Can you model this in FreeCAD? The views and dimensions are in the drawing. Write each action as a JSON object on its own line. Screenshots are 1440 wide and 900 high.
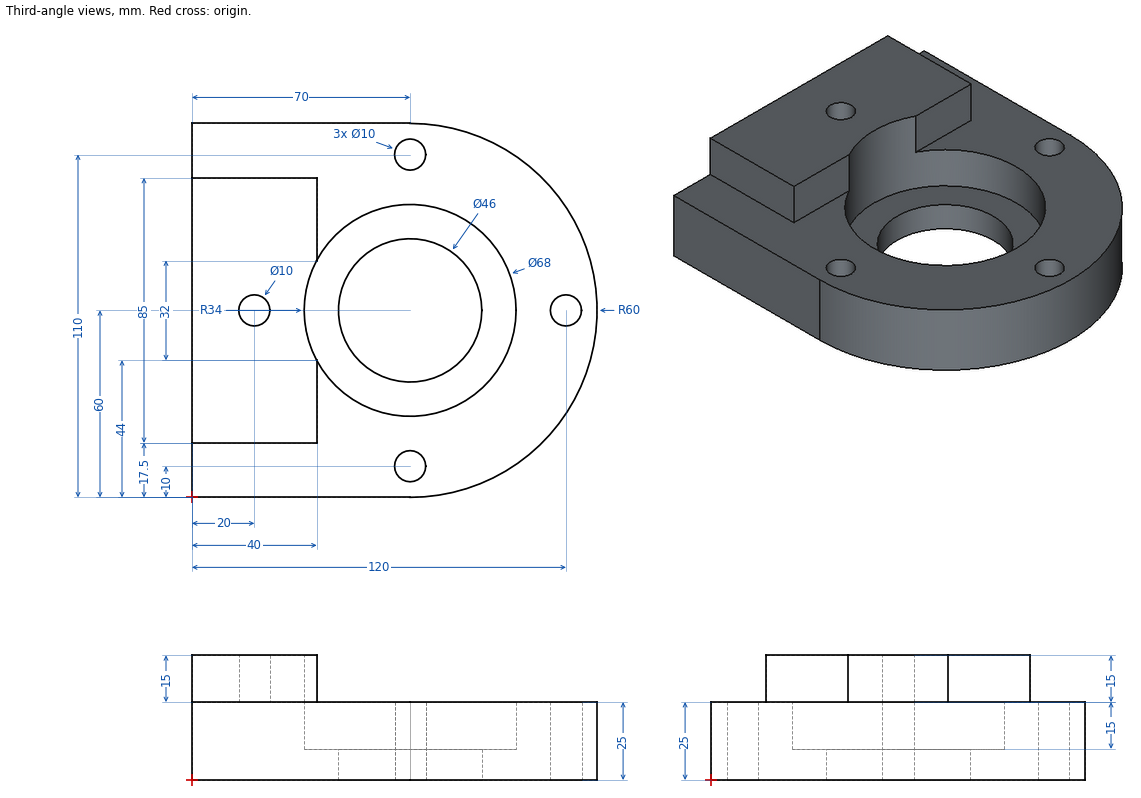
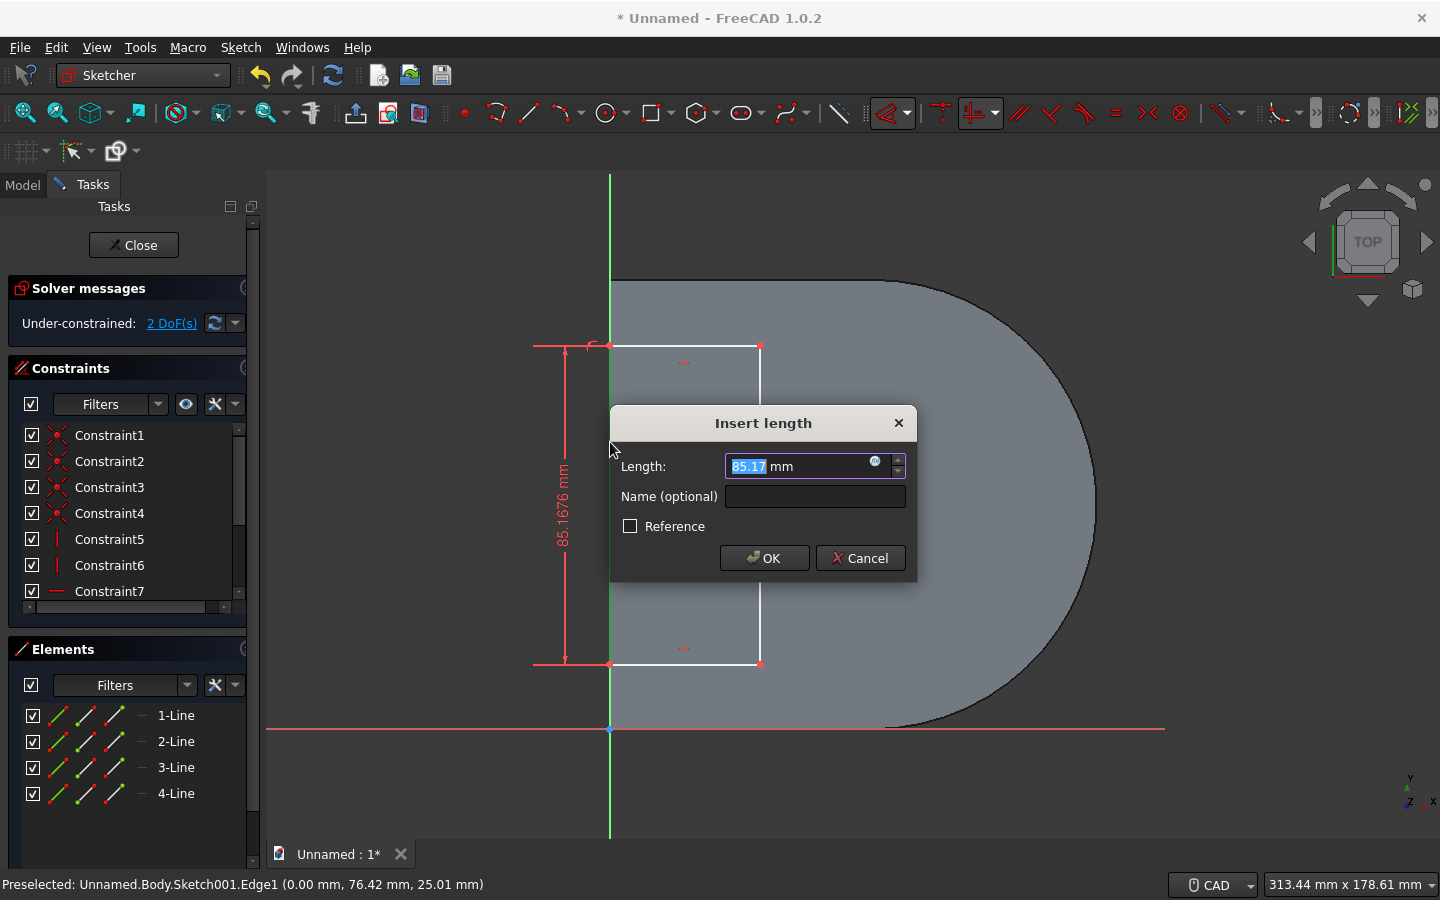
{"action": "type", "text": "85"}
{"action": "key", "text": "Return"}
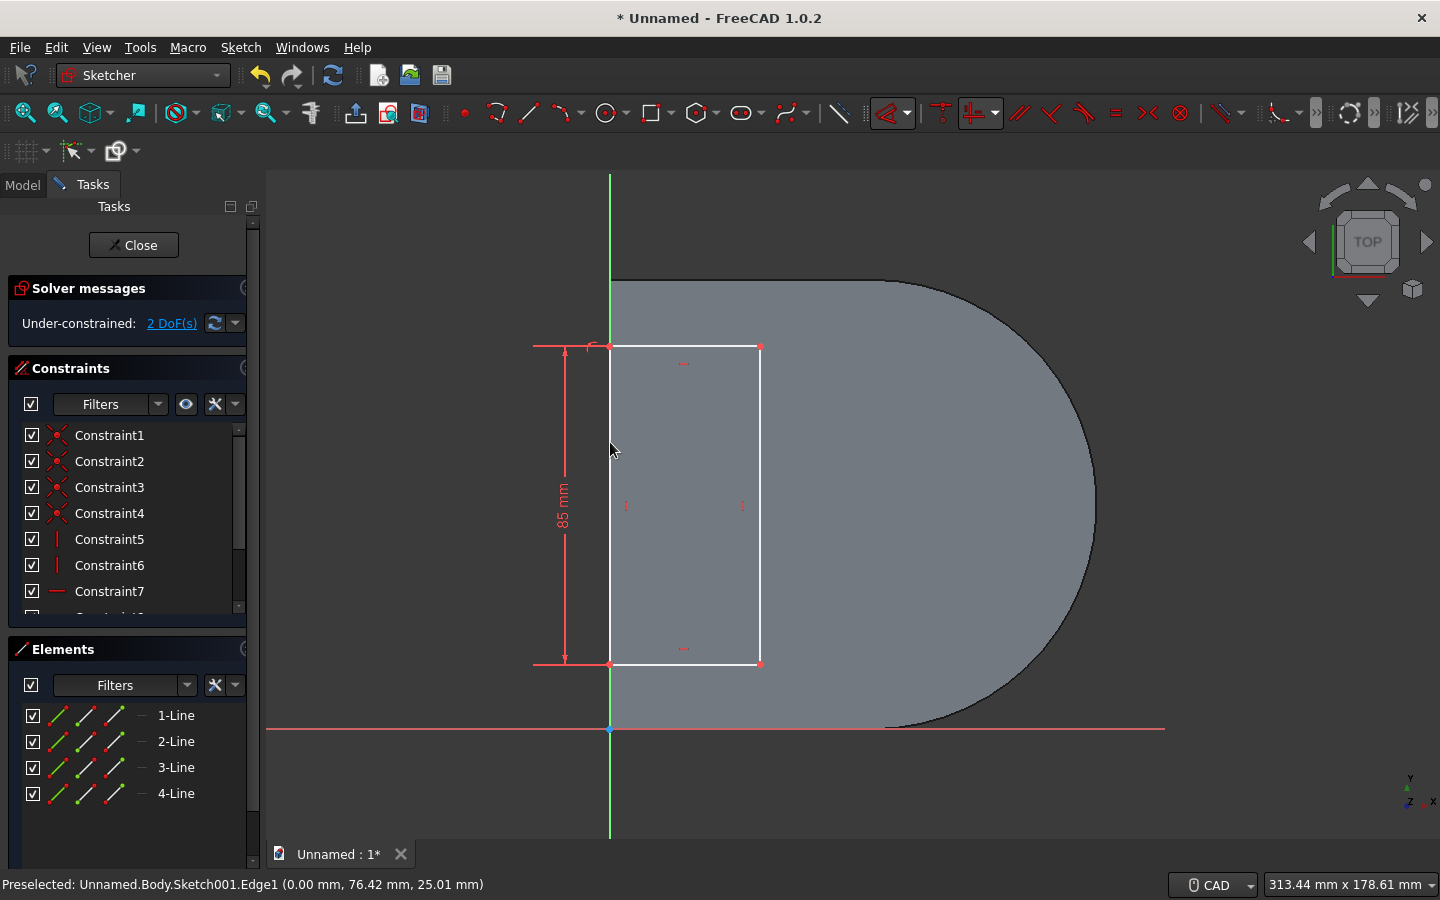
{"action": "left_click", "coordinate": [655, 665]}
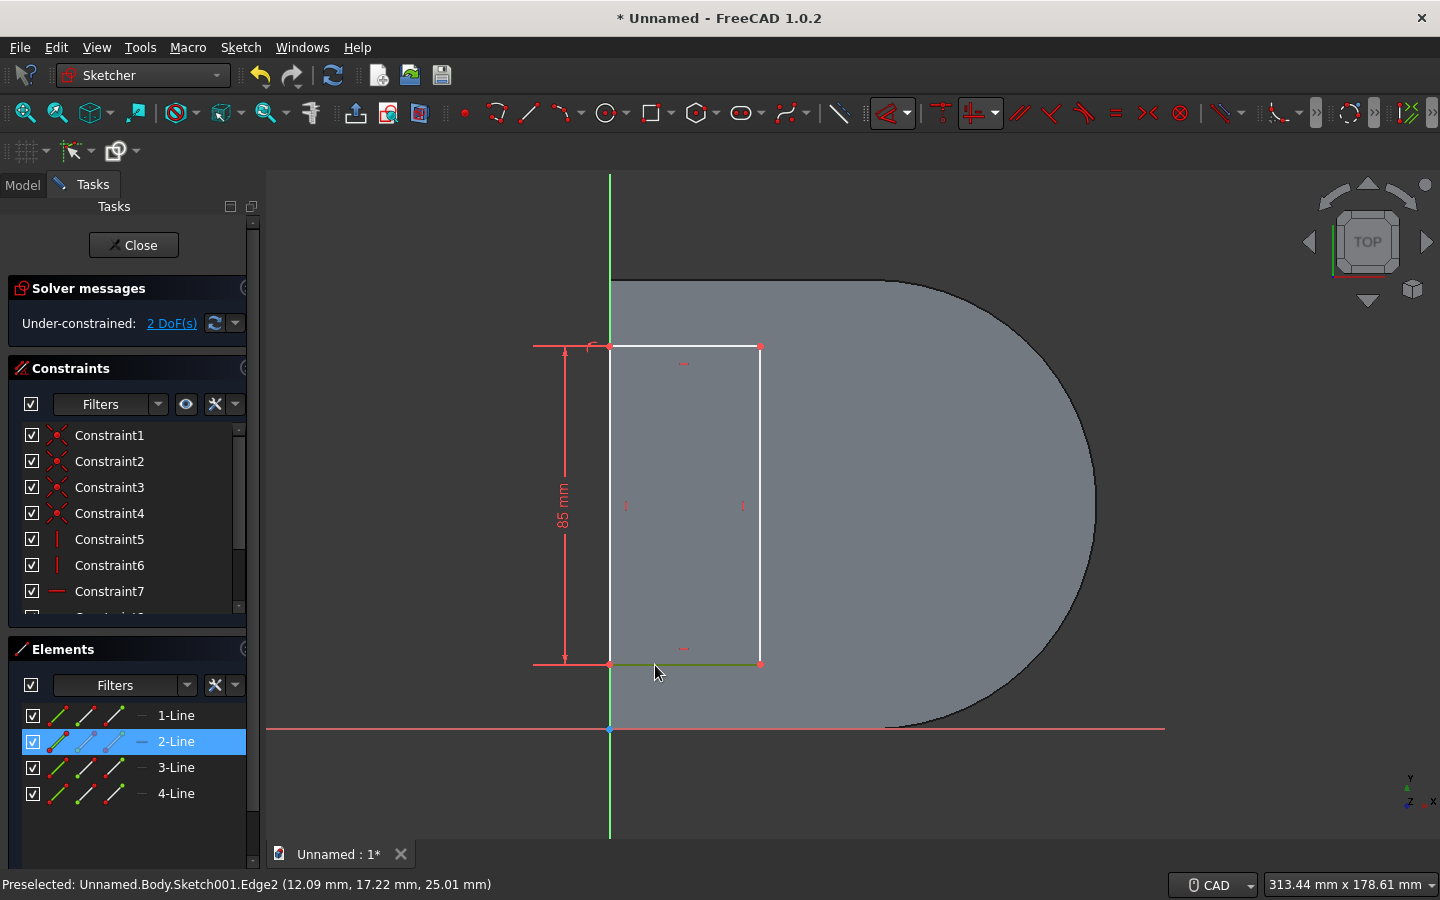
{"action": "key", "text": "l"}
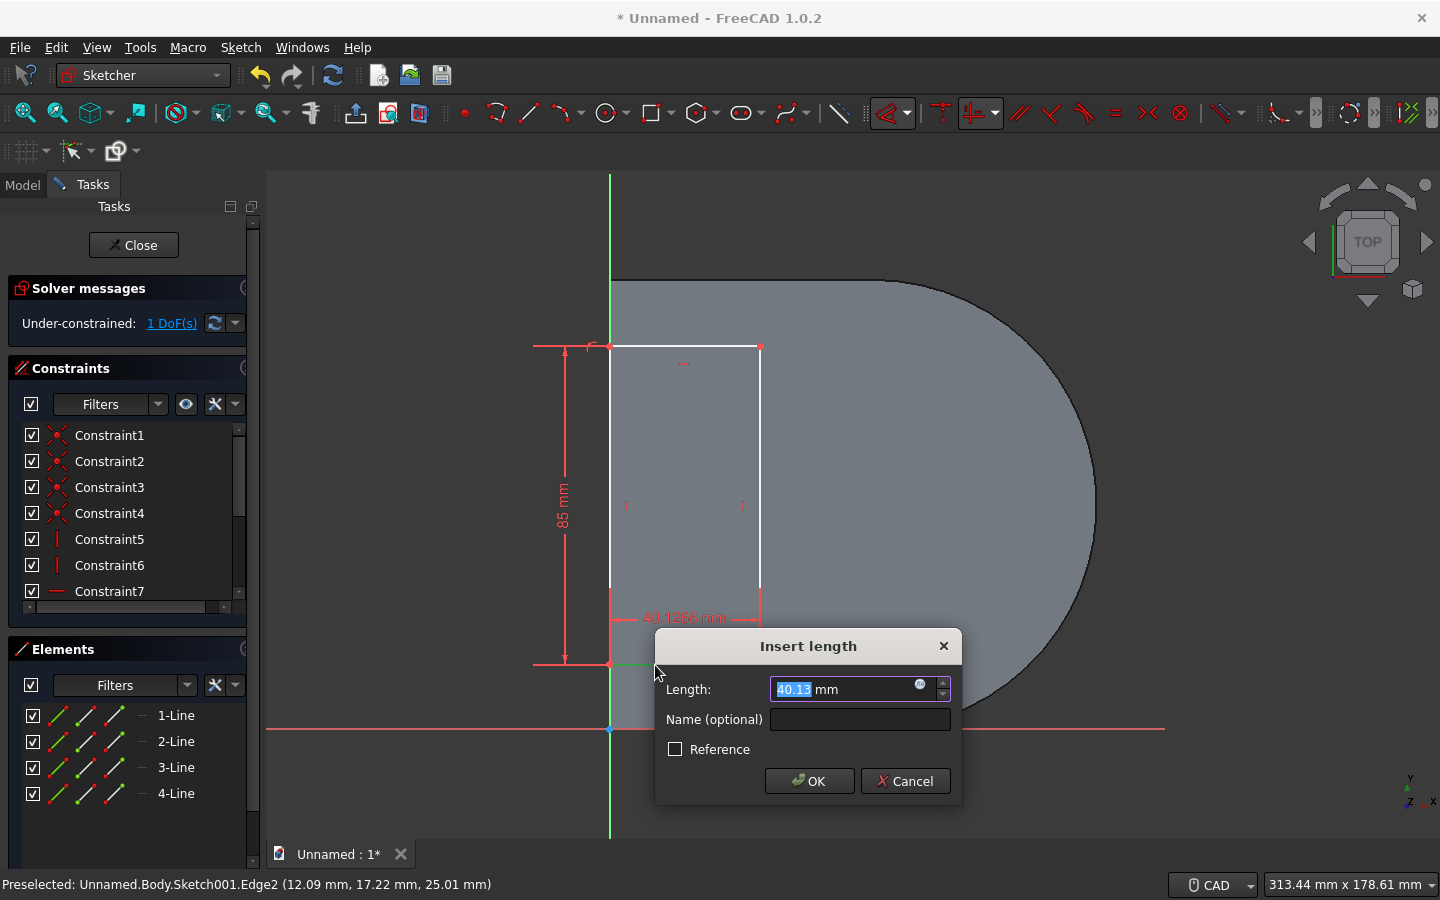
{"action": "type", "text": "40"}
{"action": "key", "text": "Return"}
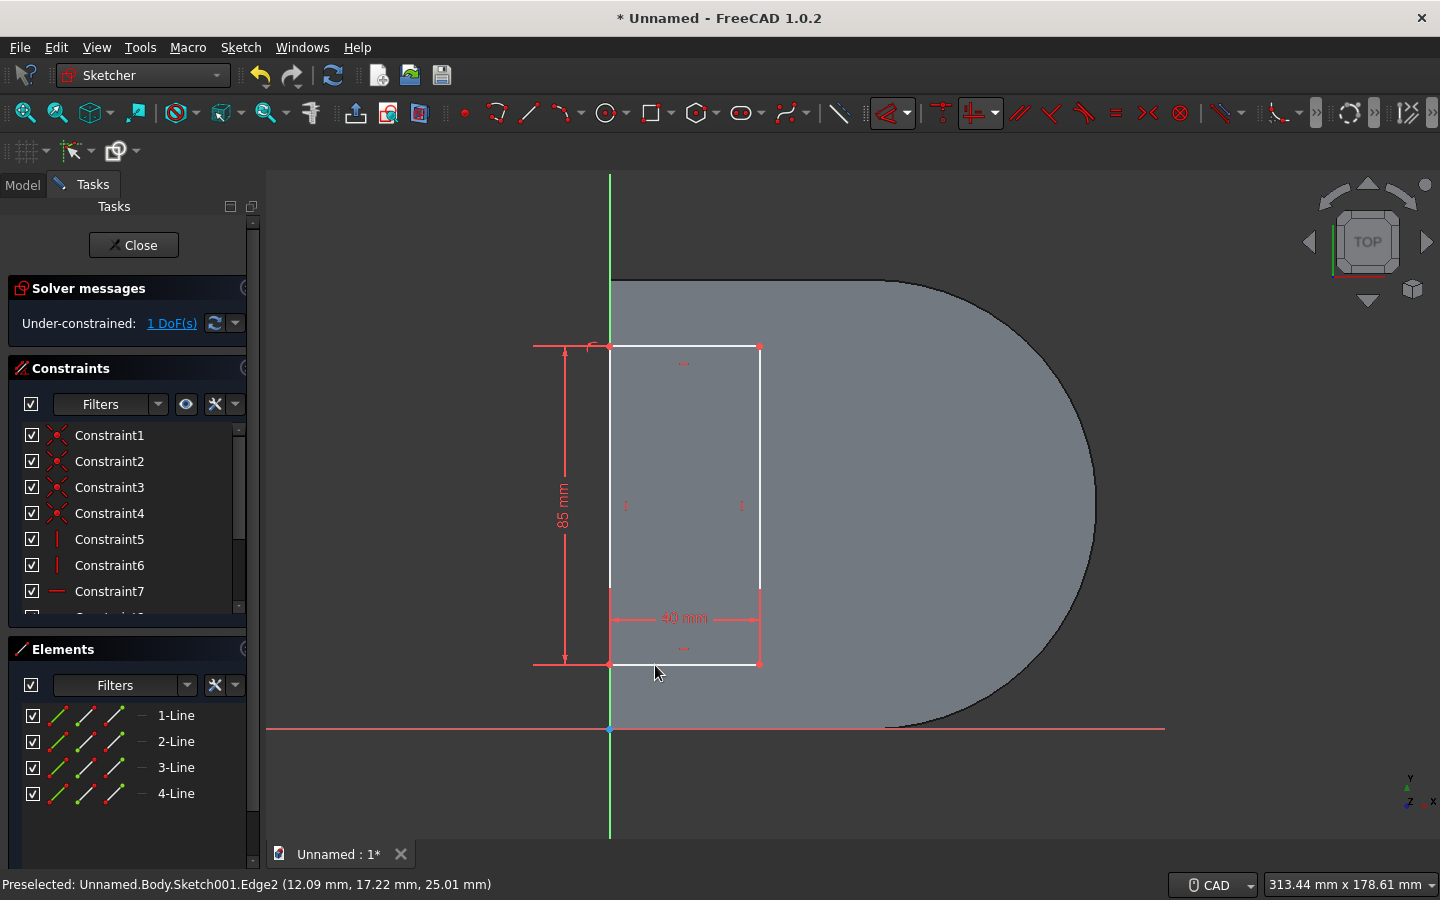
{"action": "left_click", "coordinate": [610, 665]}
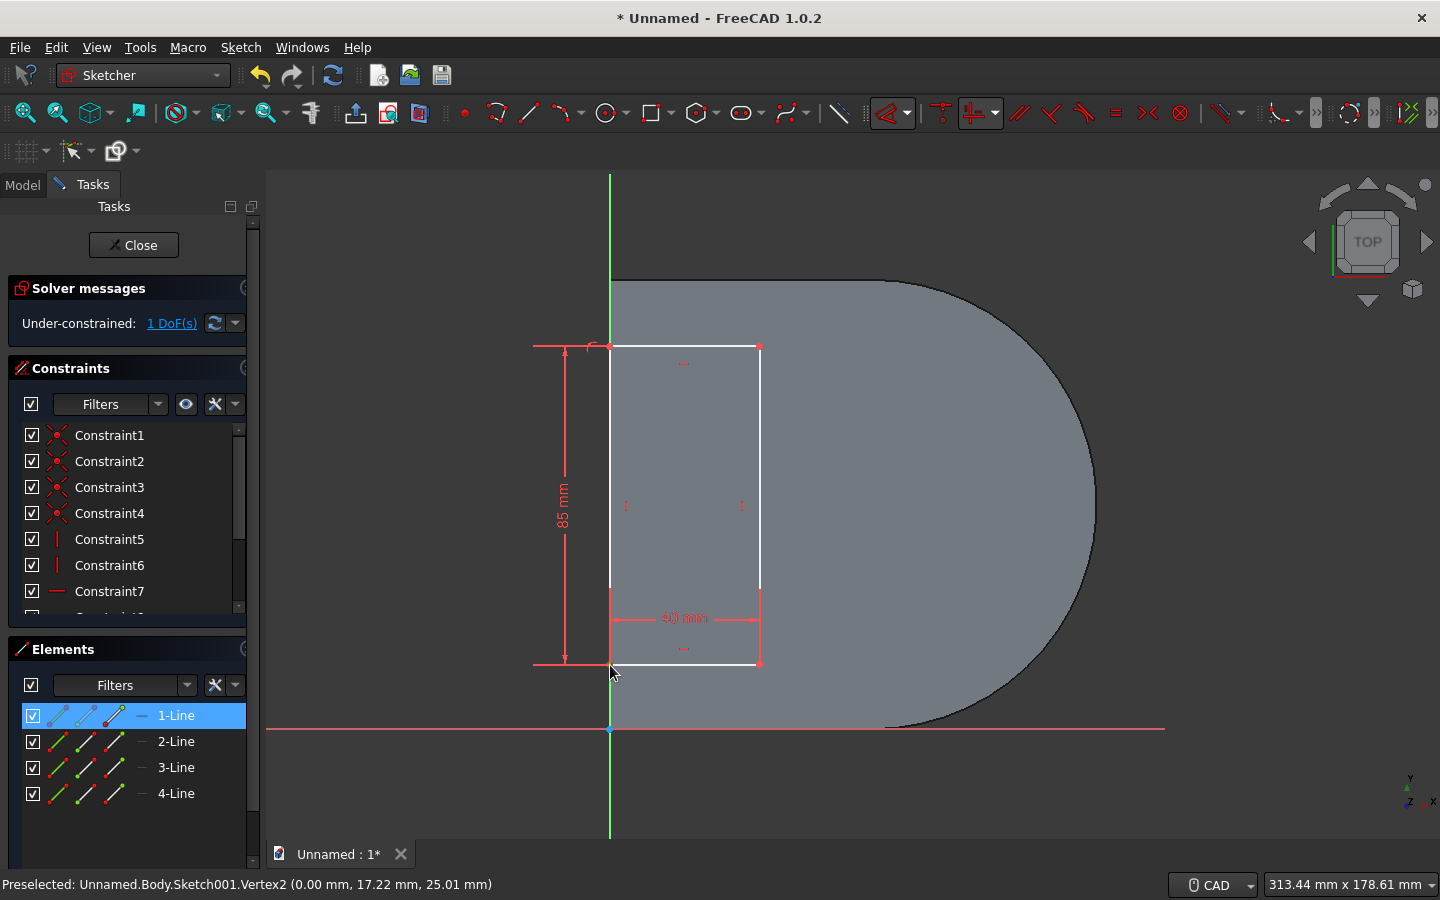
{"action": "left_click", "coordinate": [910, 114]}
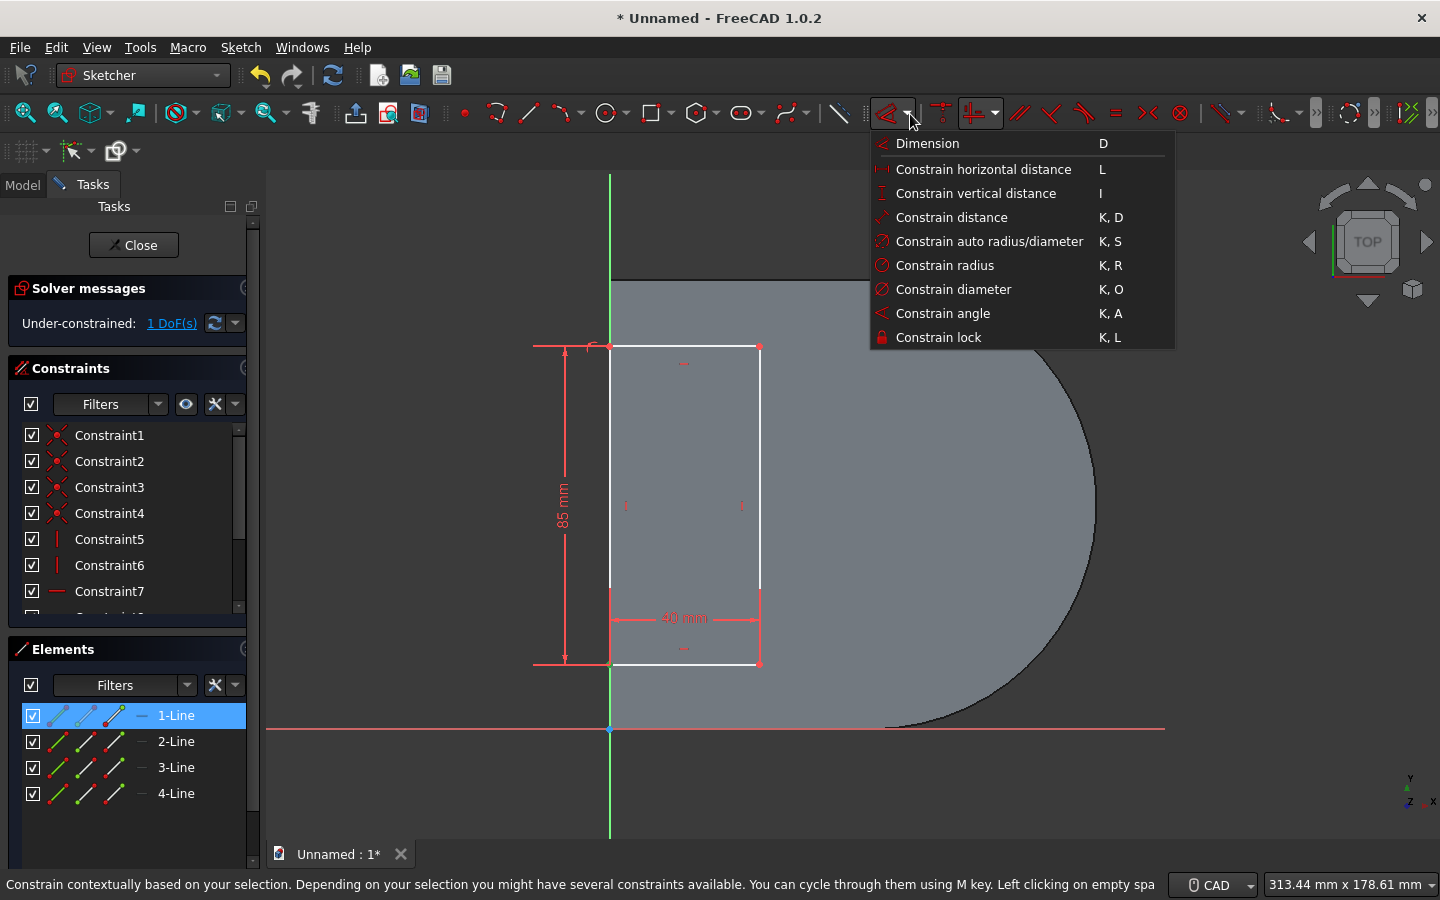
{"action": "left_click", "coordinate": [1023, 193]}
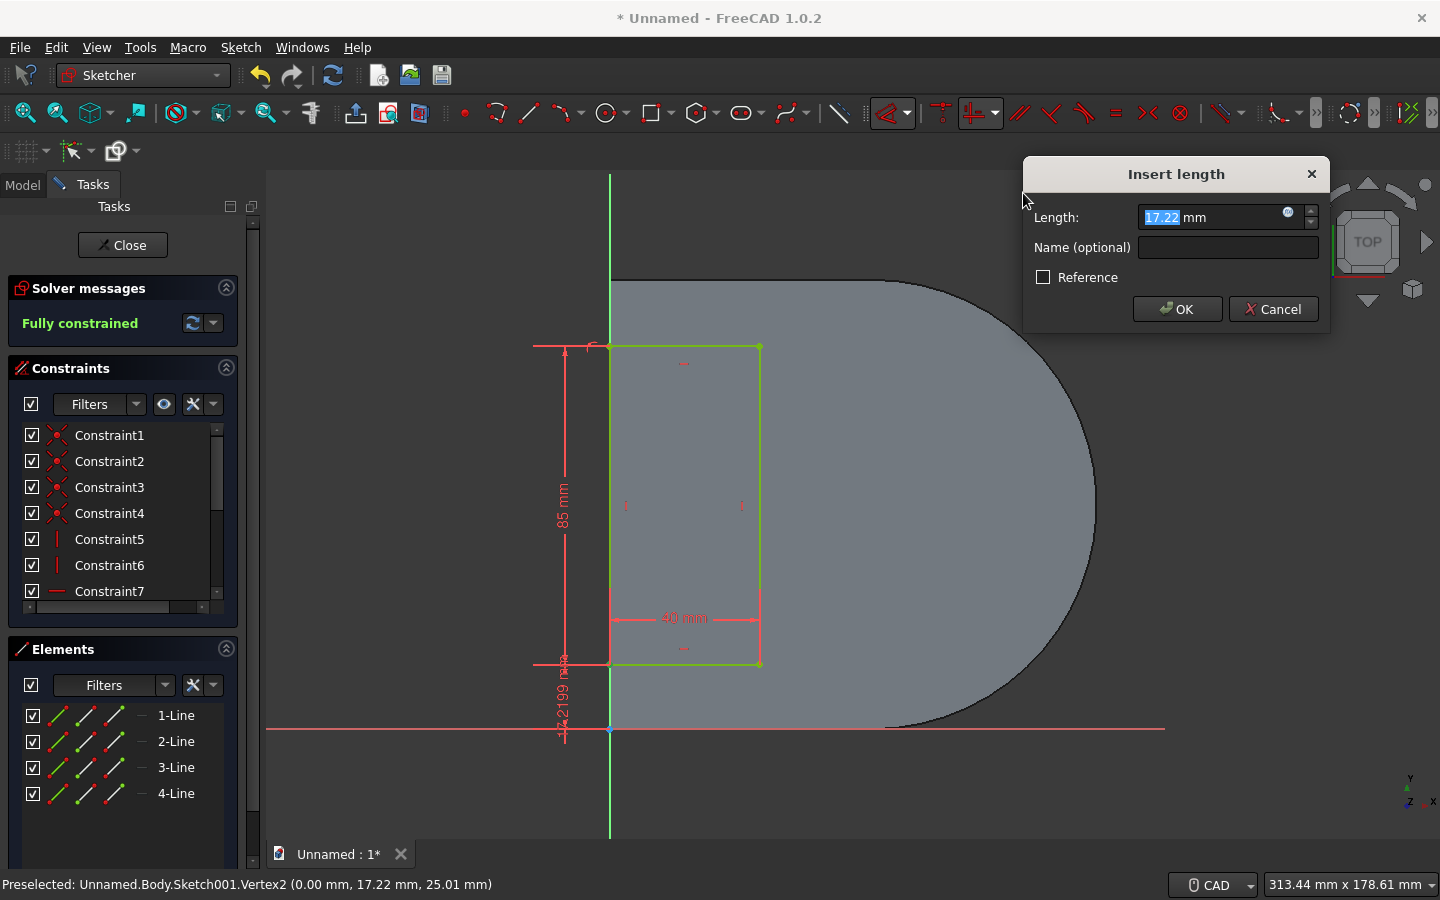
{"action": "type", "text": "17.5"}
{"action": "key", "text": "Return"}